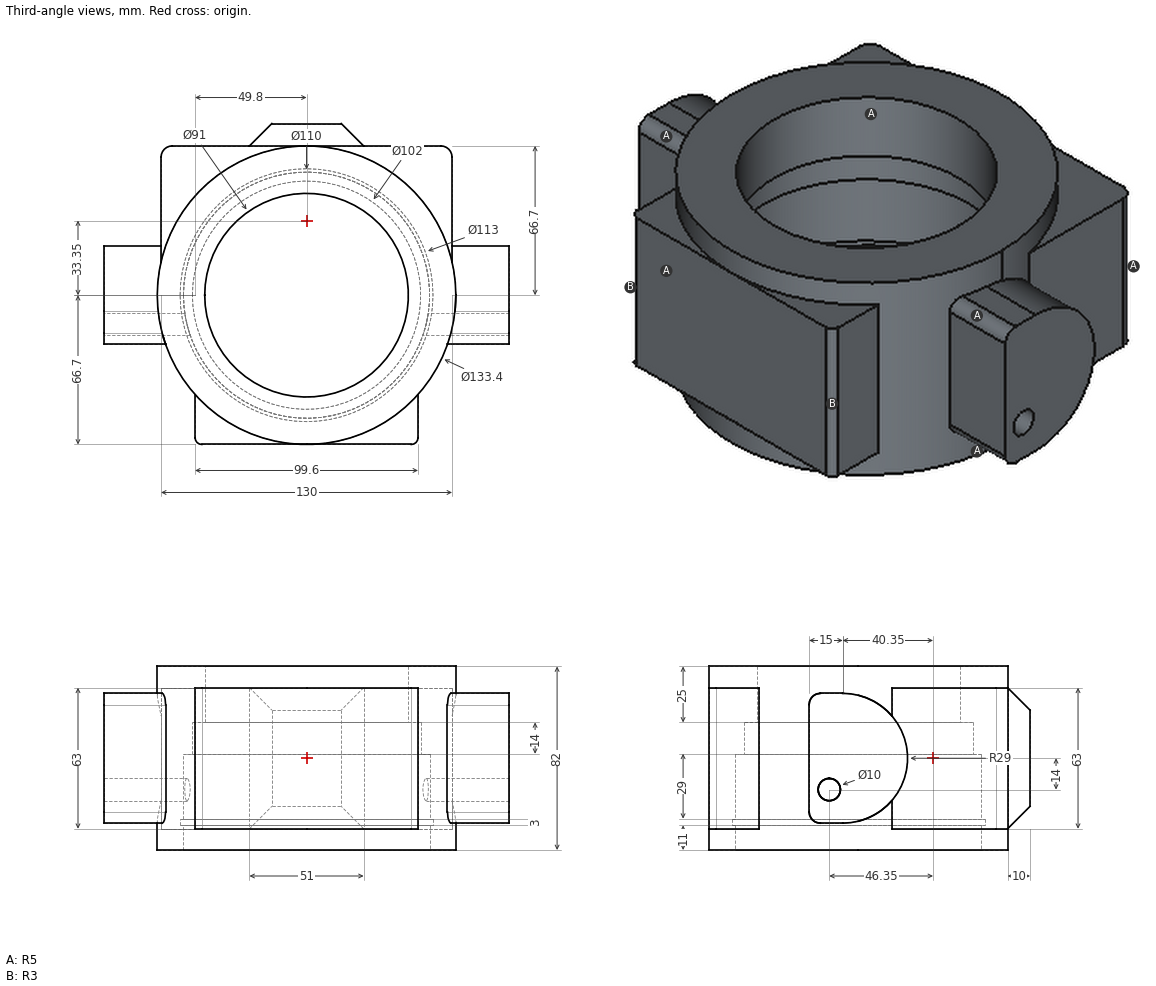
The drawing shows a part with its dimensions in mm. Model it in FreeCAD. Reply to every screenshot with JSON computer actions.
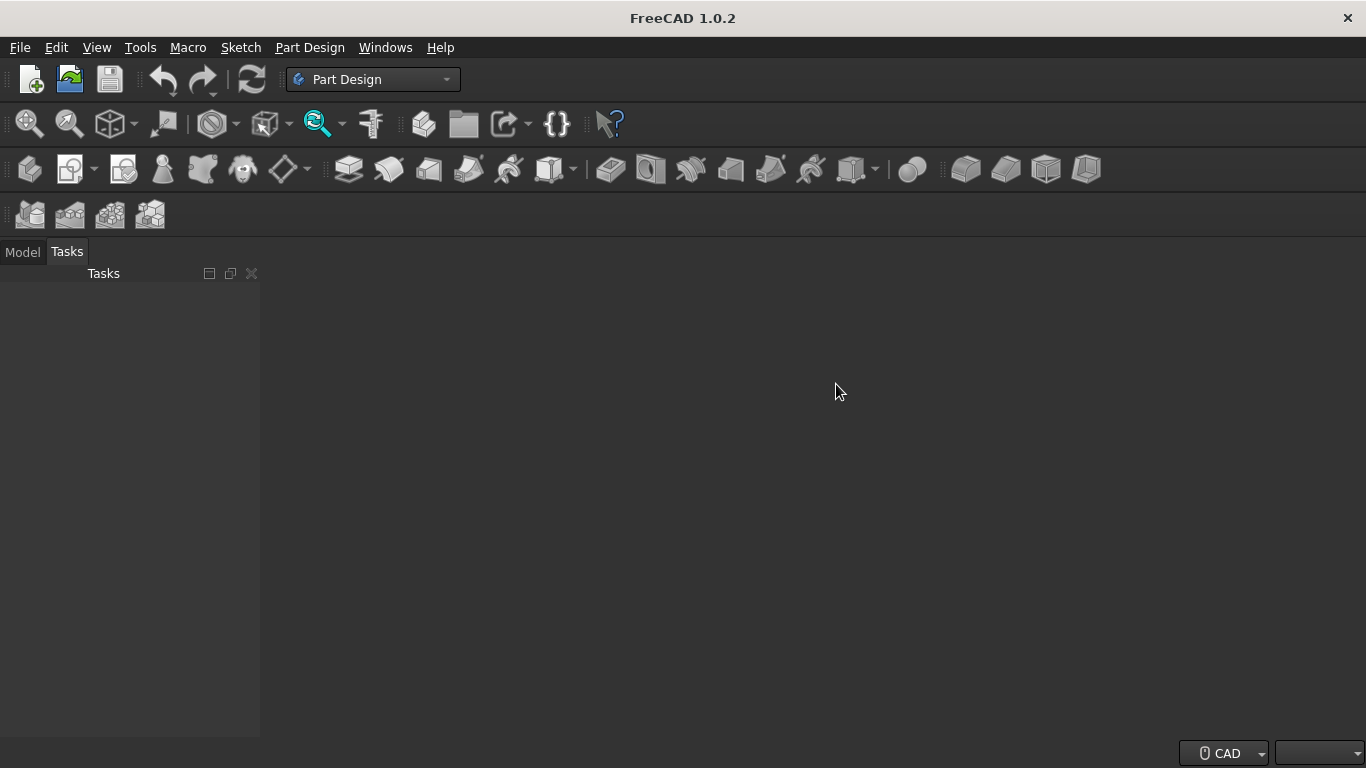
{"action": "key", "text": "ctrl+n"}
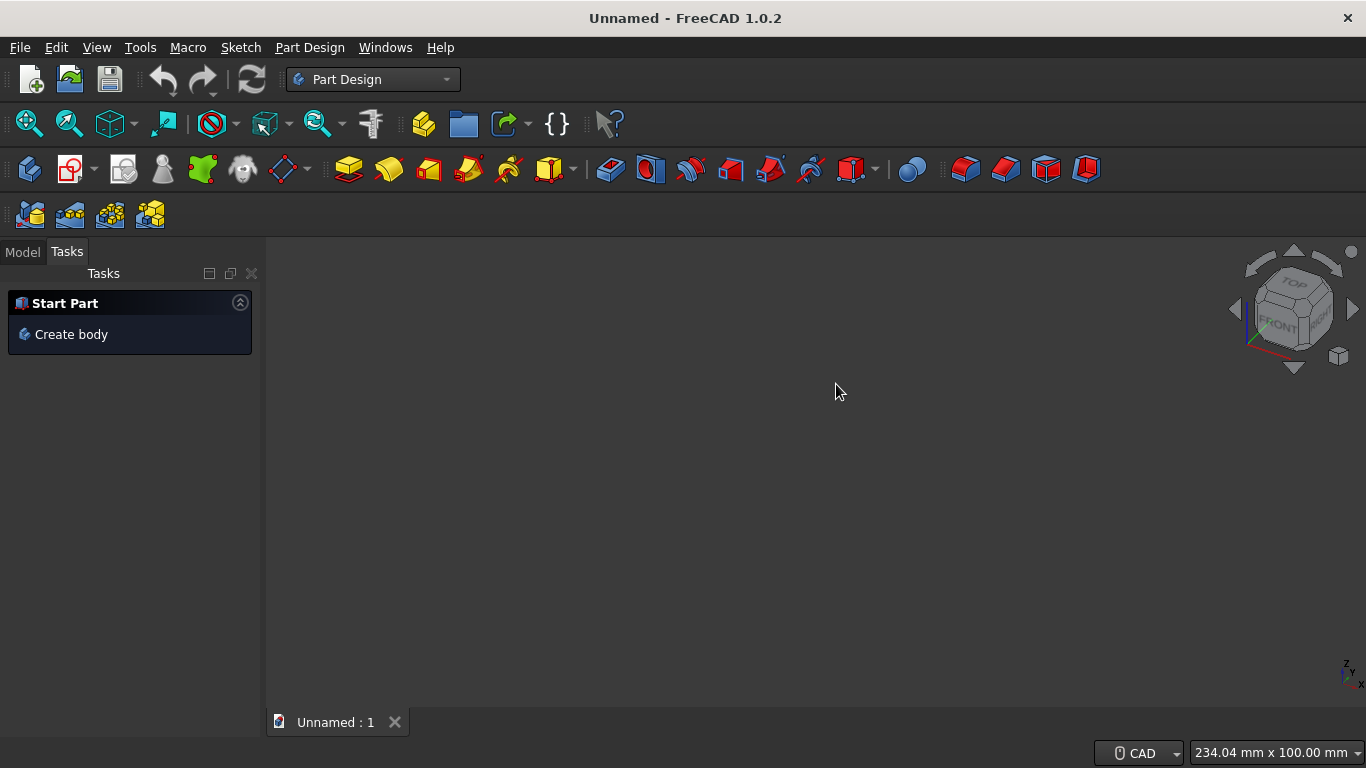
{"action": "left_click", "coordinate": [70, 170]}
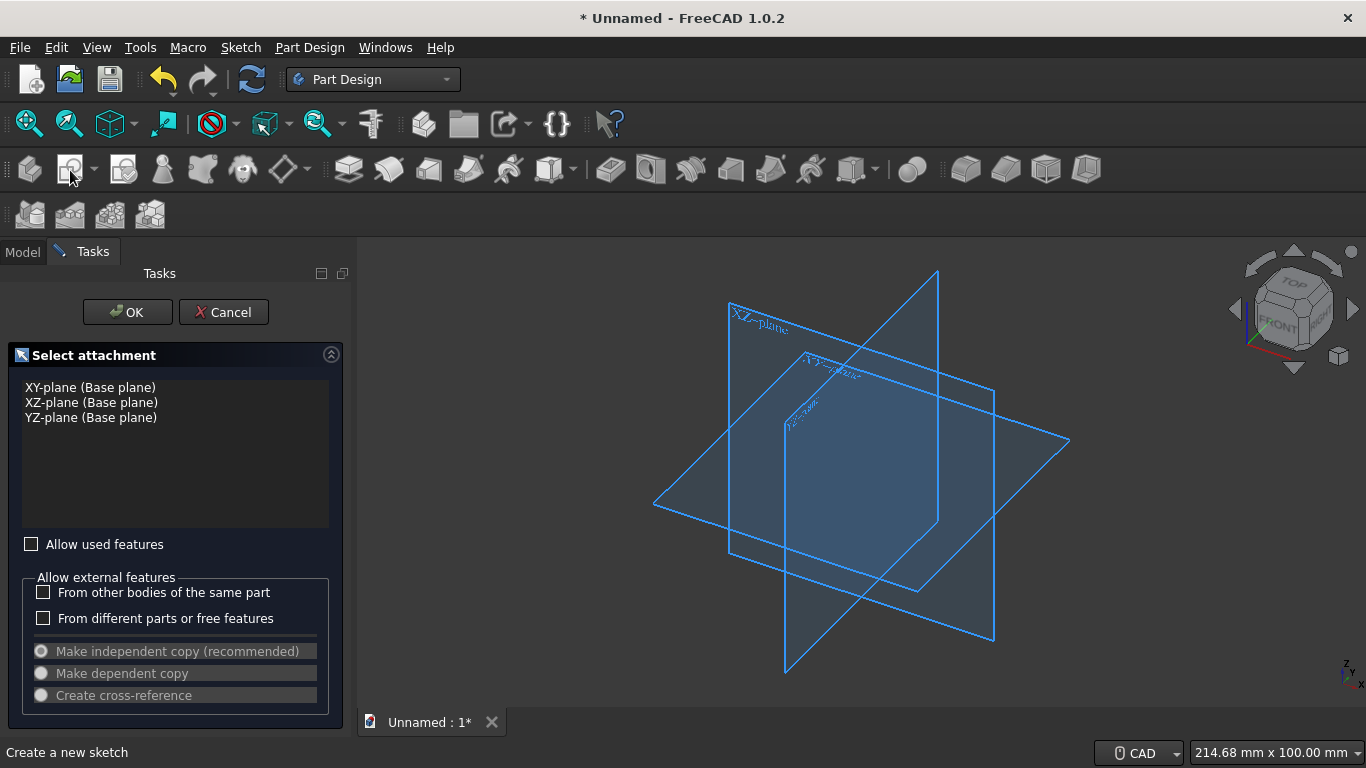
{"action": "left_click", "coordinate": [82, 388]}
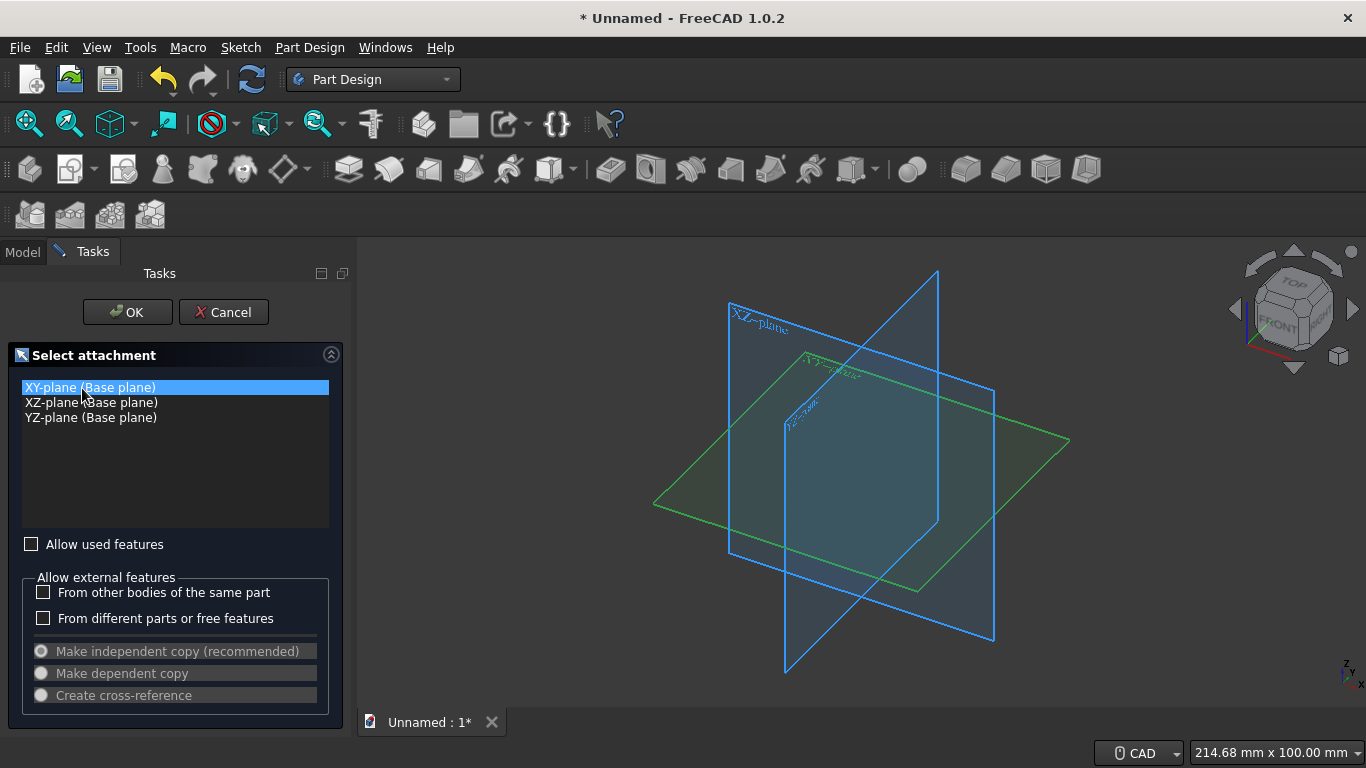
{"action": "left_click", "coordinate": [128, 312]}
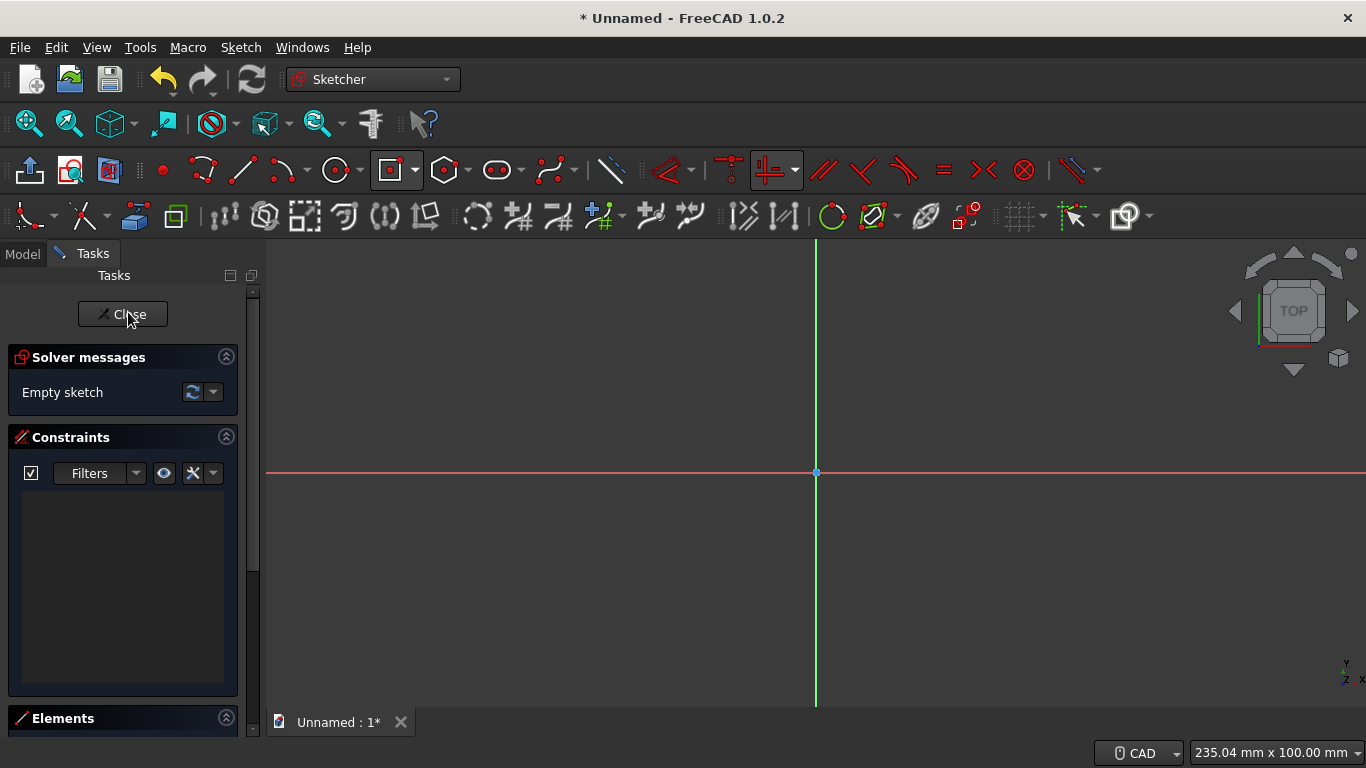
{"action": "key", "text": "g v"}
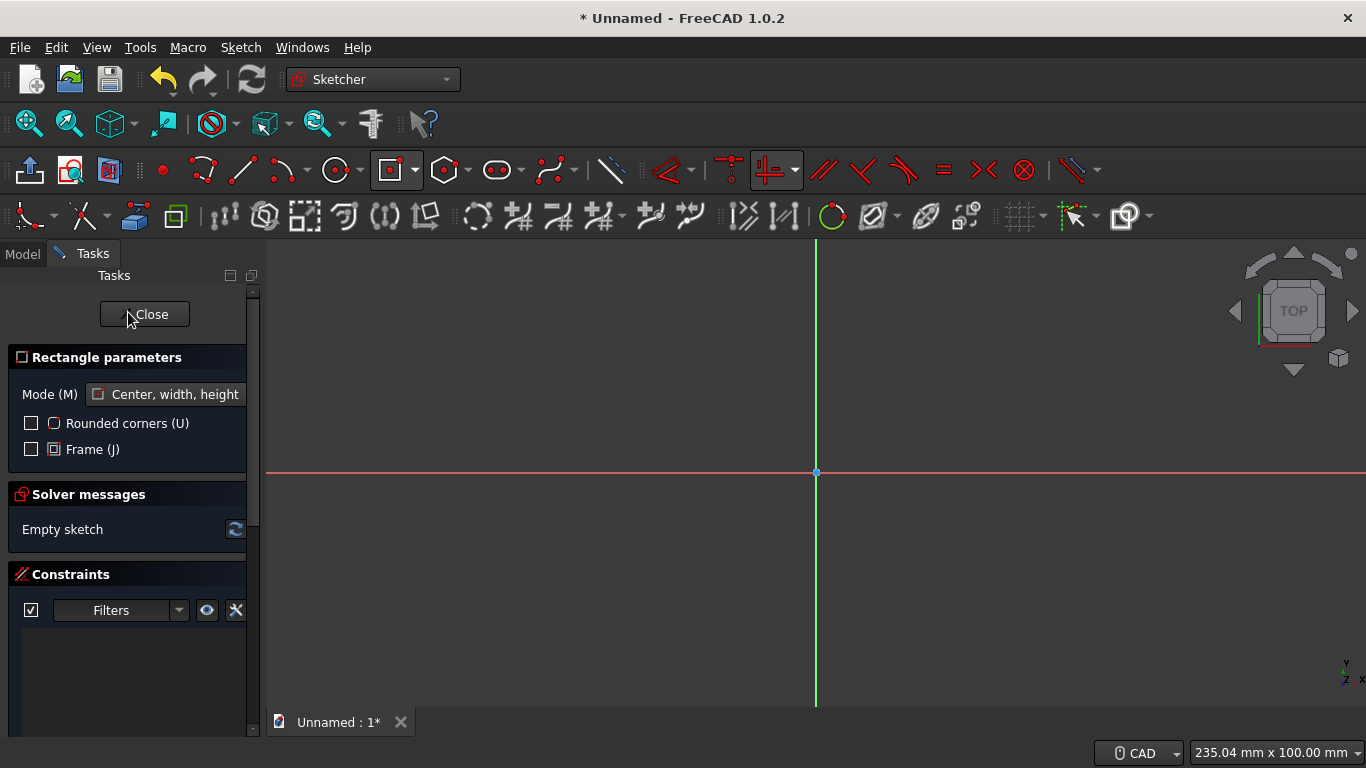
{"action": "left_click", "coordinate": [816, 473]}
{"action": "left_click", "coordinate": [1120, 317]}
{"action": "key", "text": "Escape"}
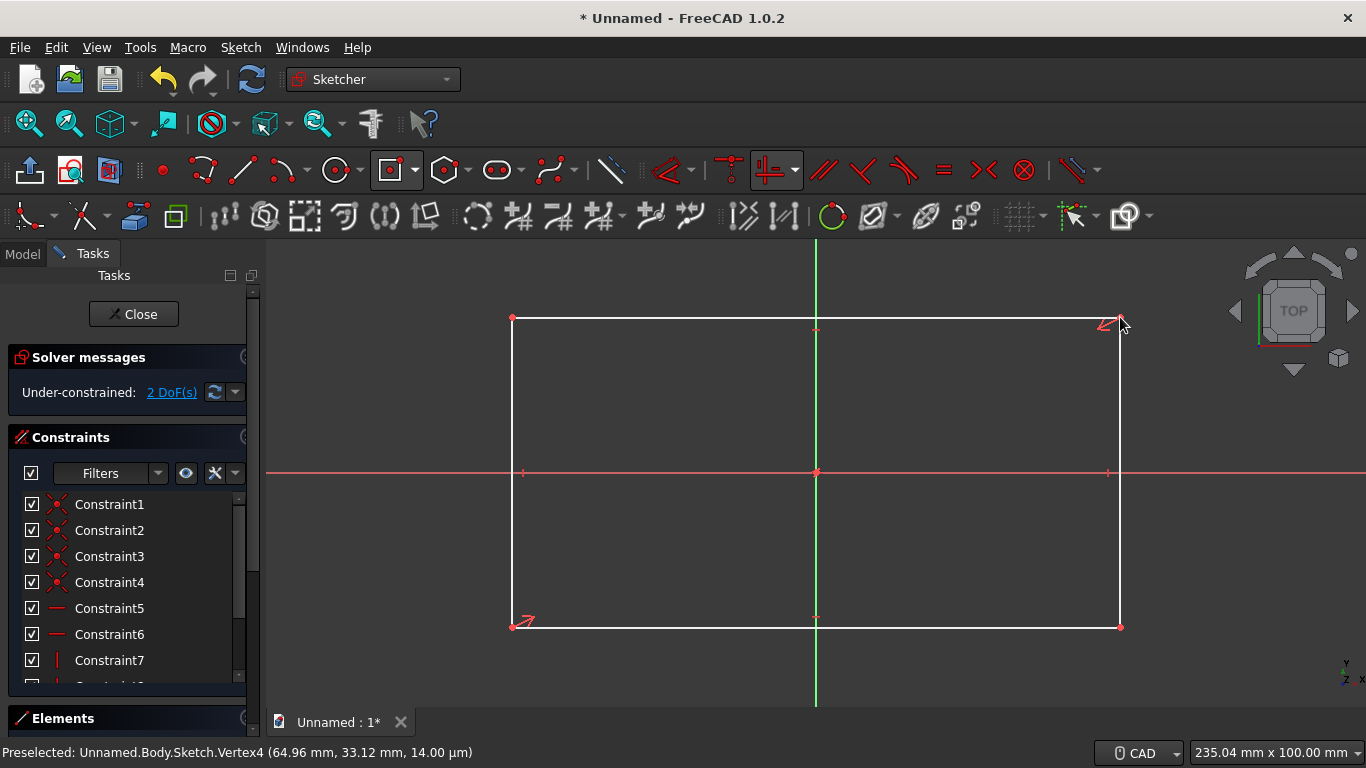
{"action": "left_click", "coordinate": [666, 170]}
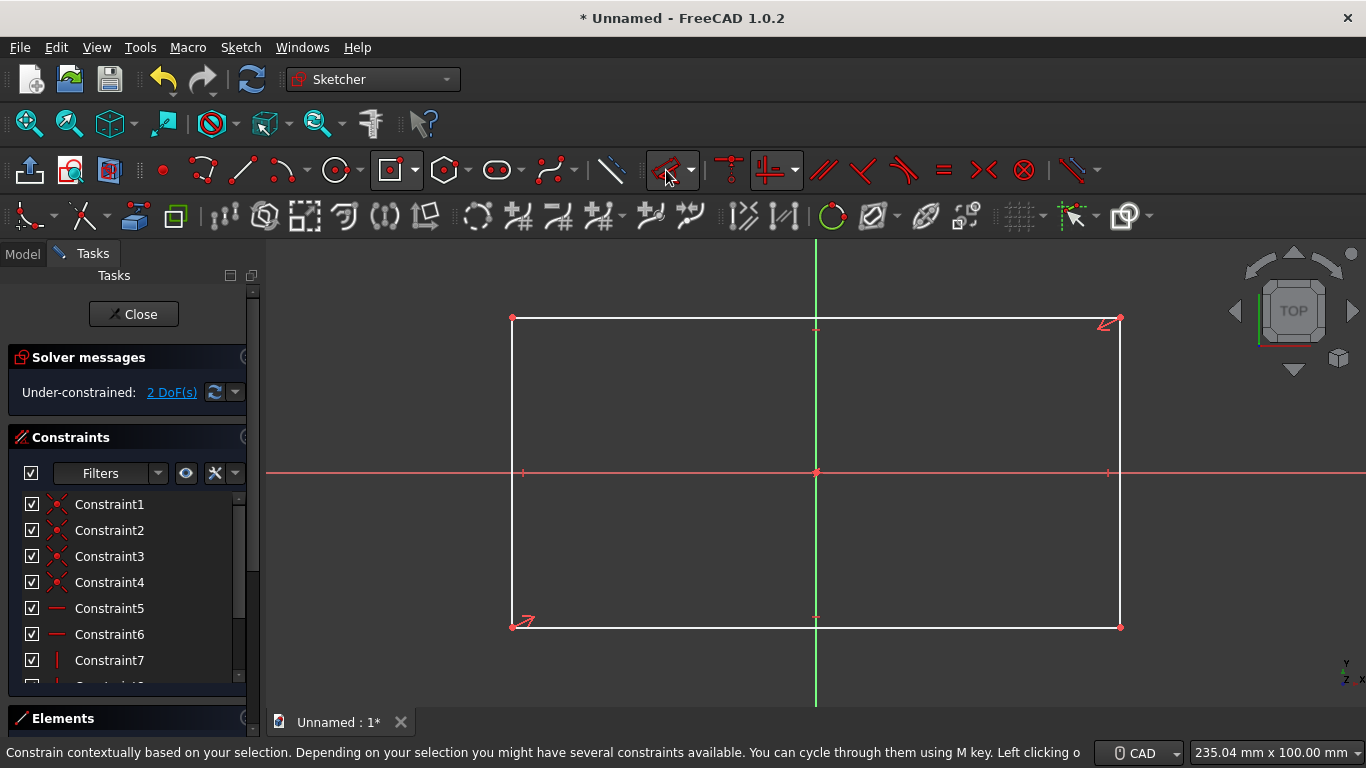
{"action": "left_click", "coordinate": [694, 628]}
{"action": "left_click", "coordinate": [676, 662]}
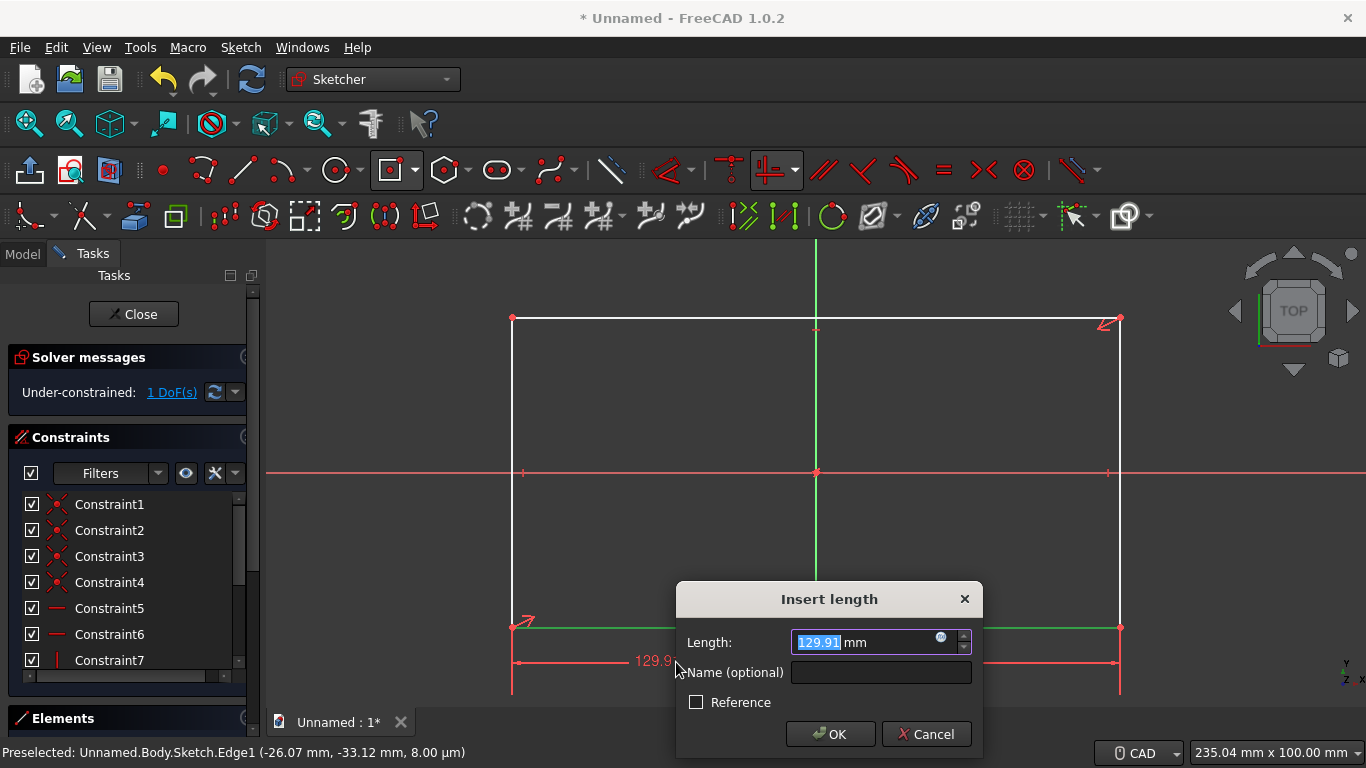
{"action": "type", "text": "130"}
{"action": "key", "text": "Return"}